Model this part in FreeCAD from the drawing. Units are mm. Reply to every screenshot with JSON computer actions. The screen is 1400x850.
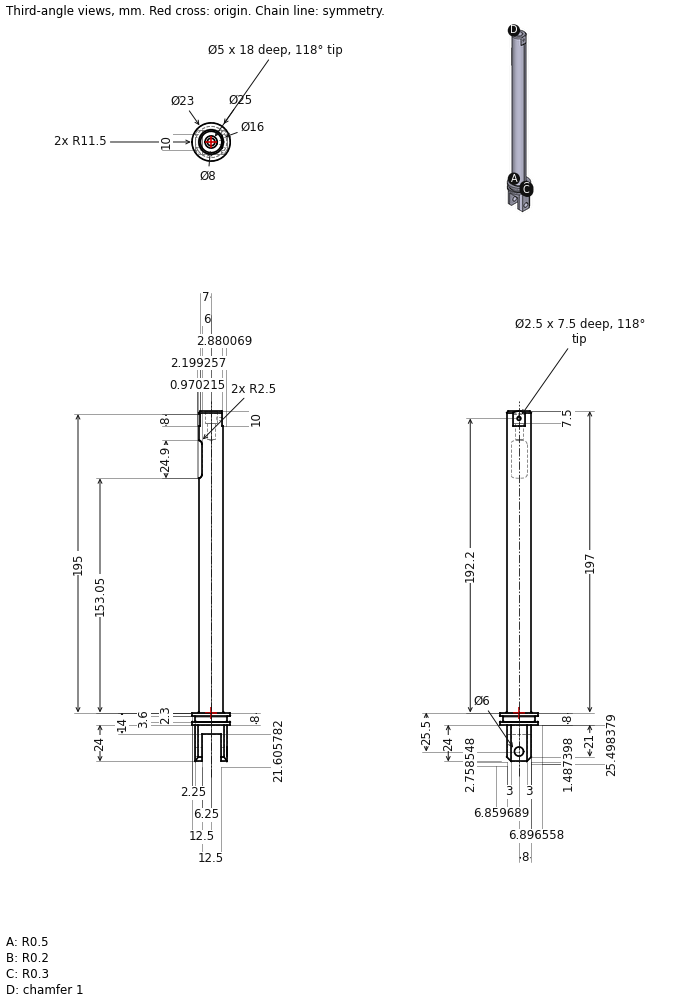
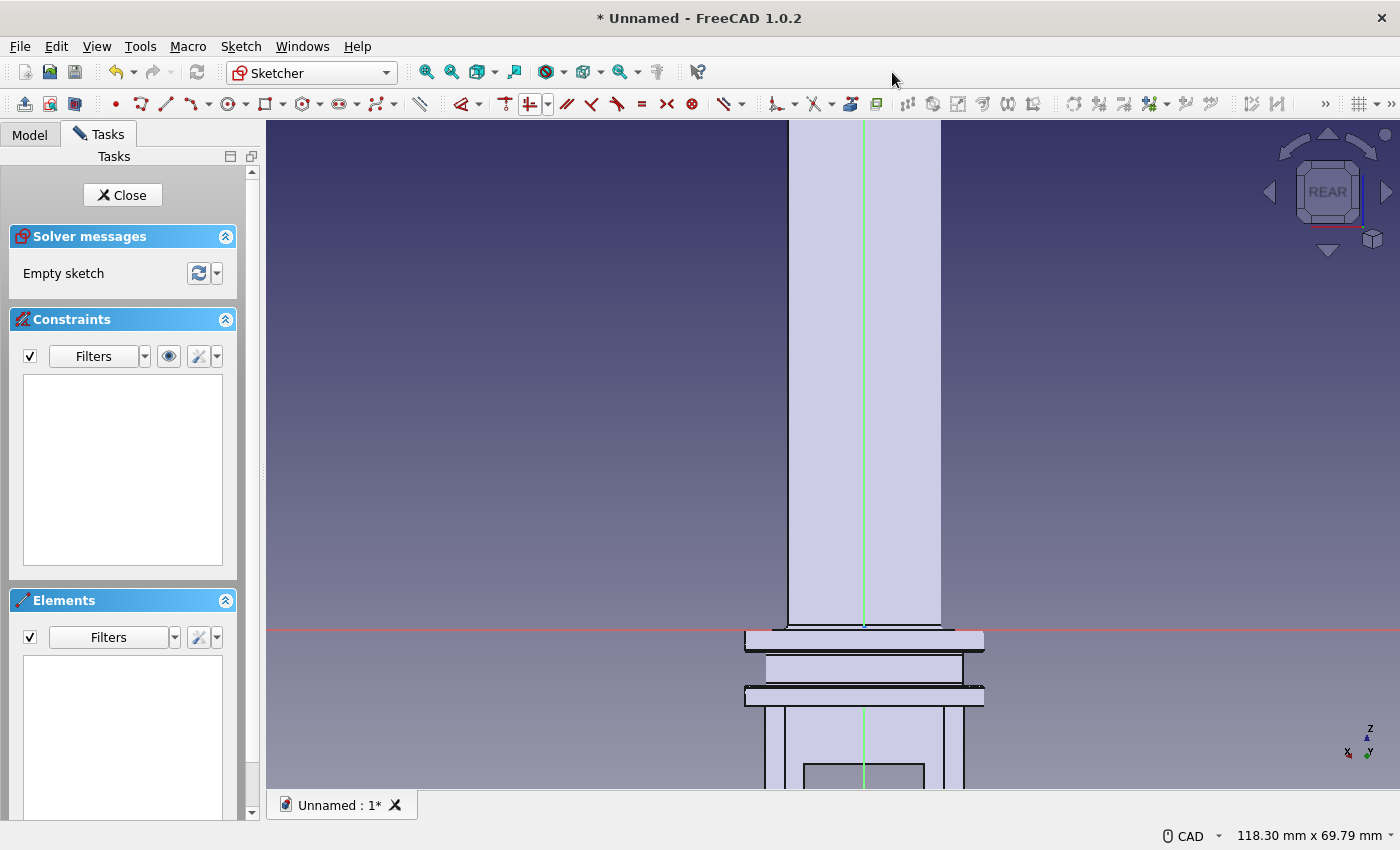
{"action": "scroll", "coordinate": [764, 454], "scroll_direction": "down", "scroll_amount": 5}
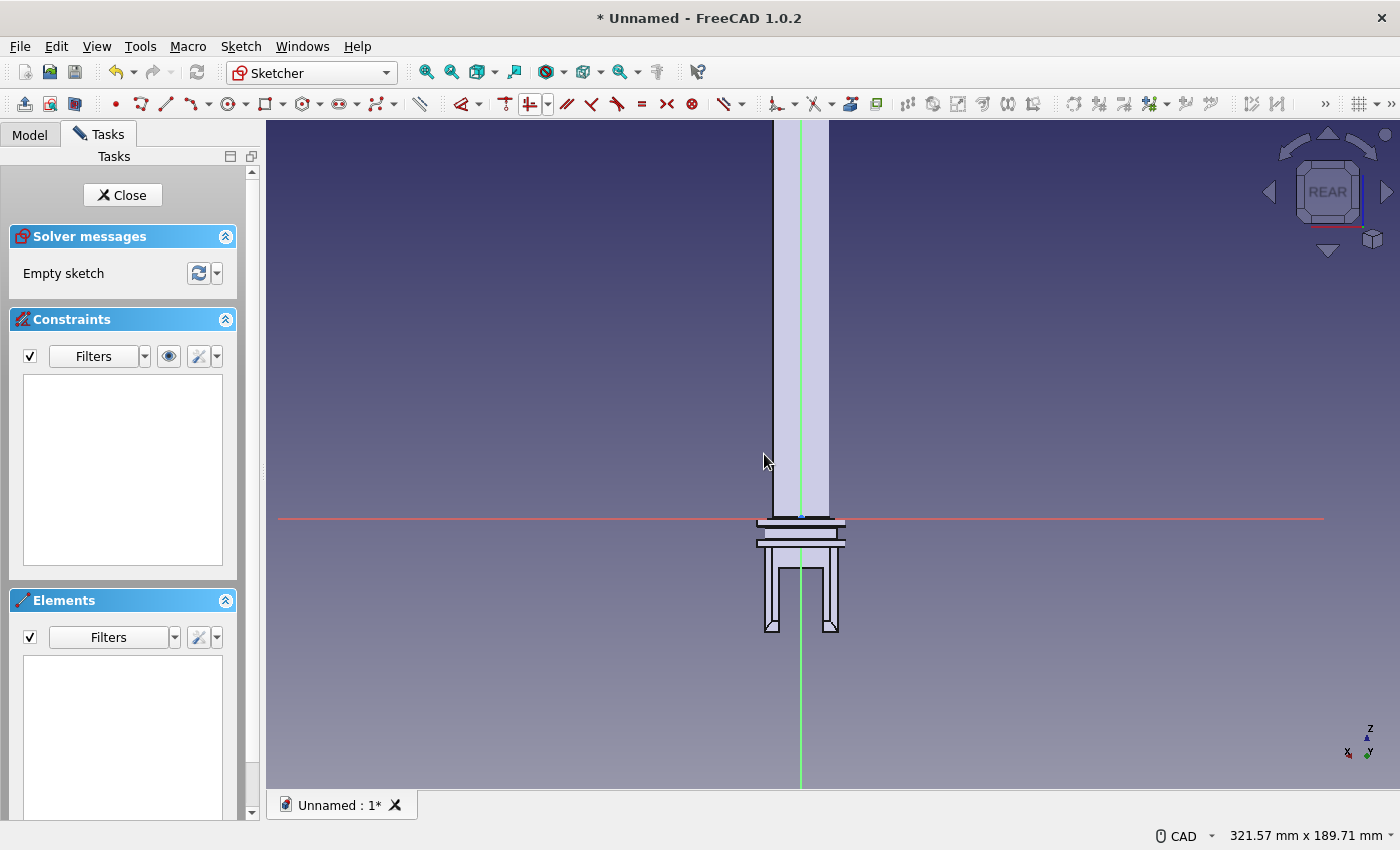
{"action": "scroll", "coordinate": [764, 454], "scroll_direction": "down", "scroll_amount": 5}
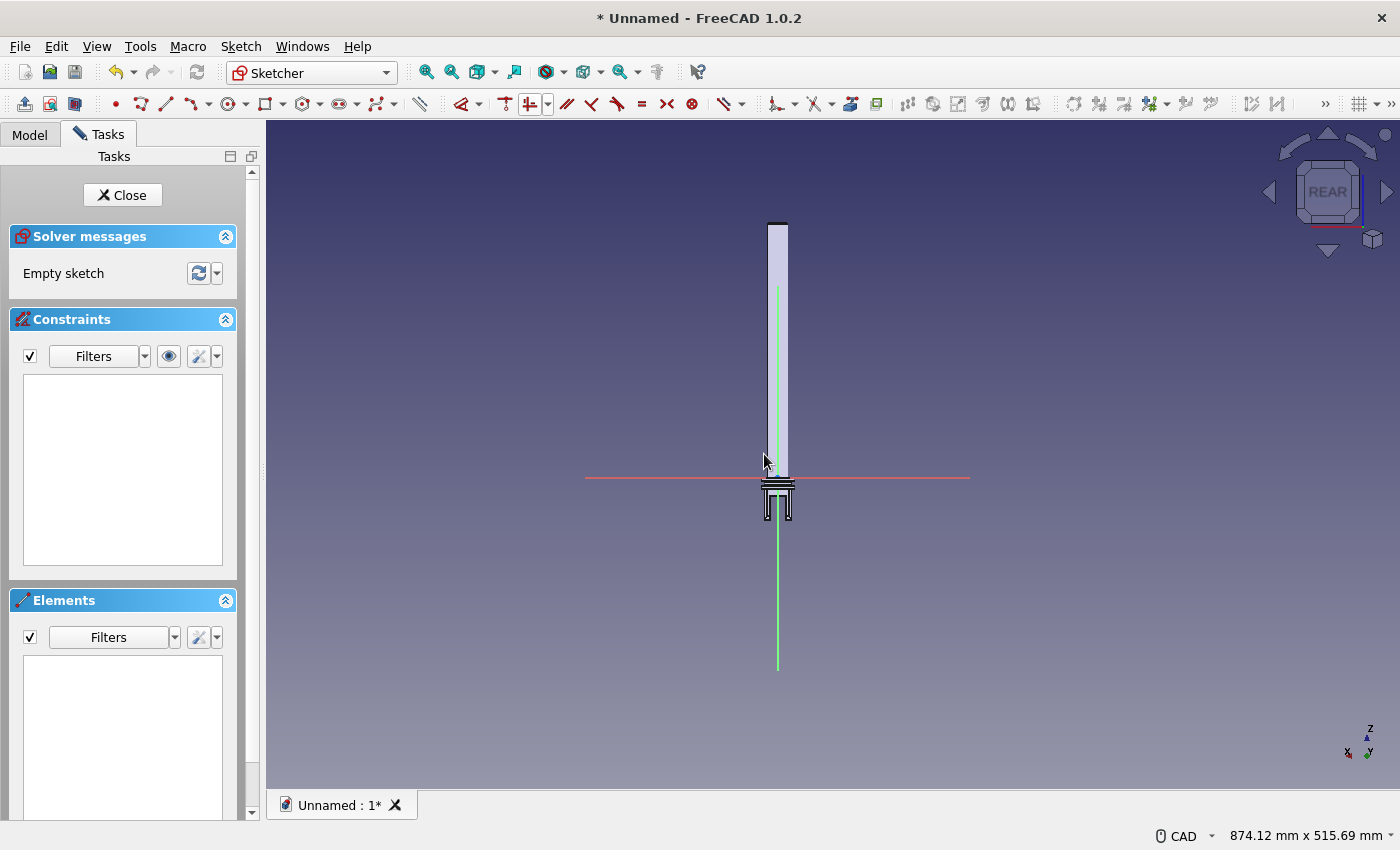
{"action": "scroll", "coordinate": [780, 219], "scroll_direction": "up", "scroll_amount": 10}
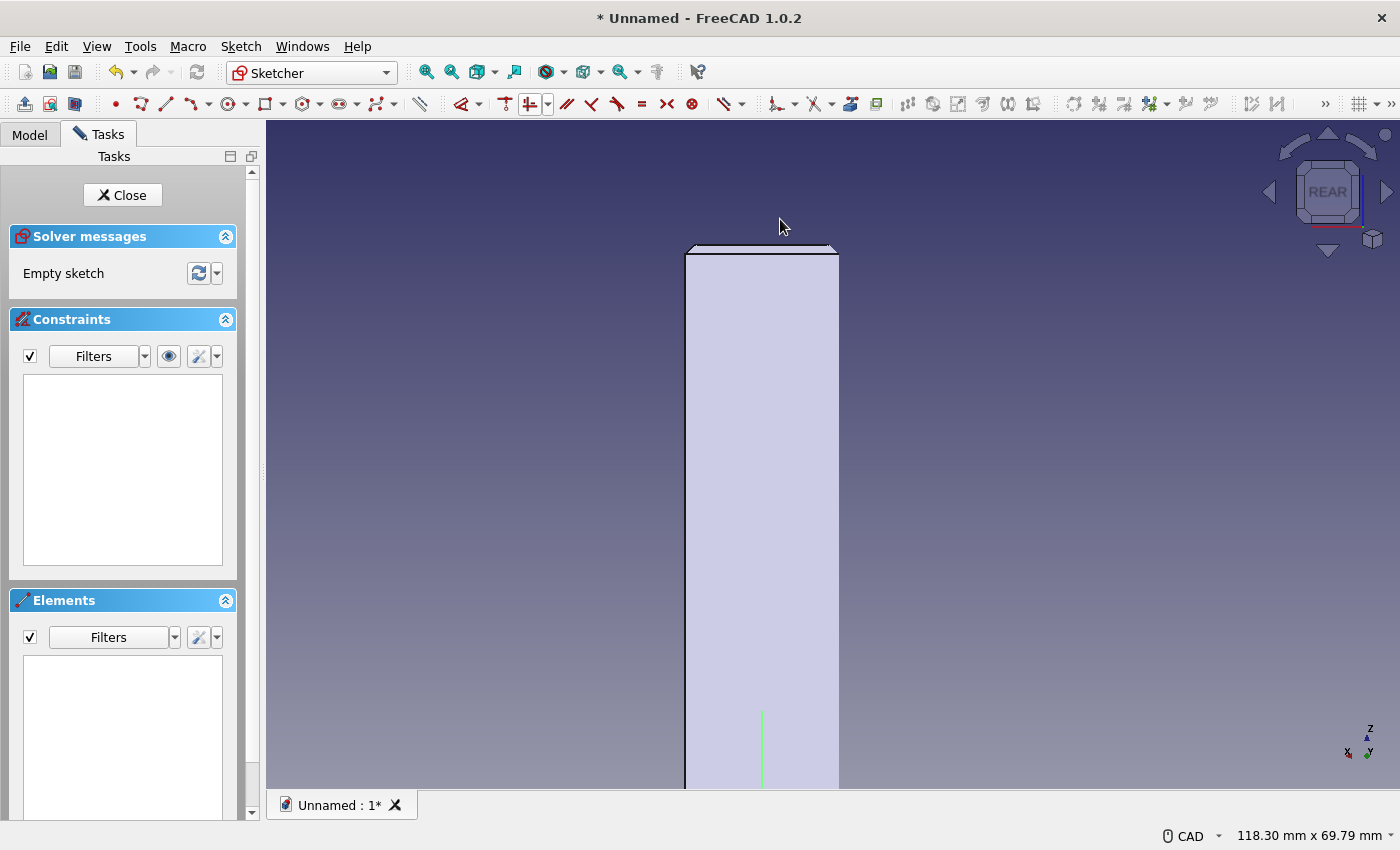
{"action": "left_click", "coordinate": [264, 104]}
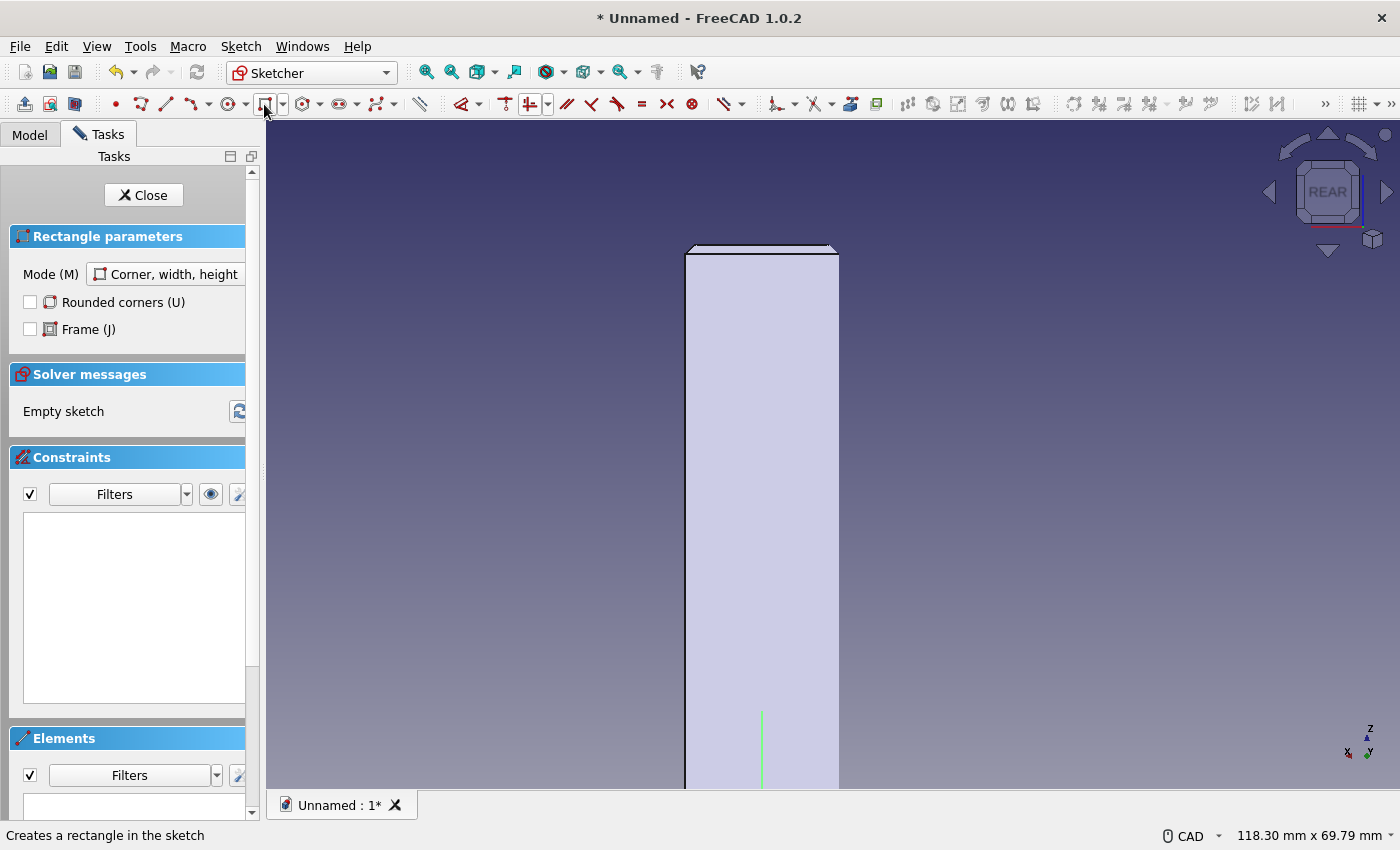
{"action": "left_click", "coordinate": [829, 264]}
{"action": "mouse_move", "coordinate": [850, 341]}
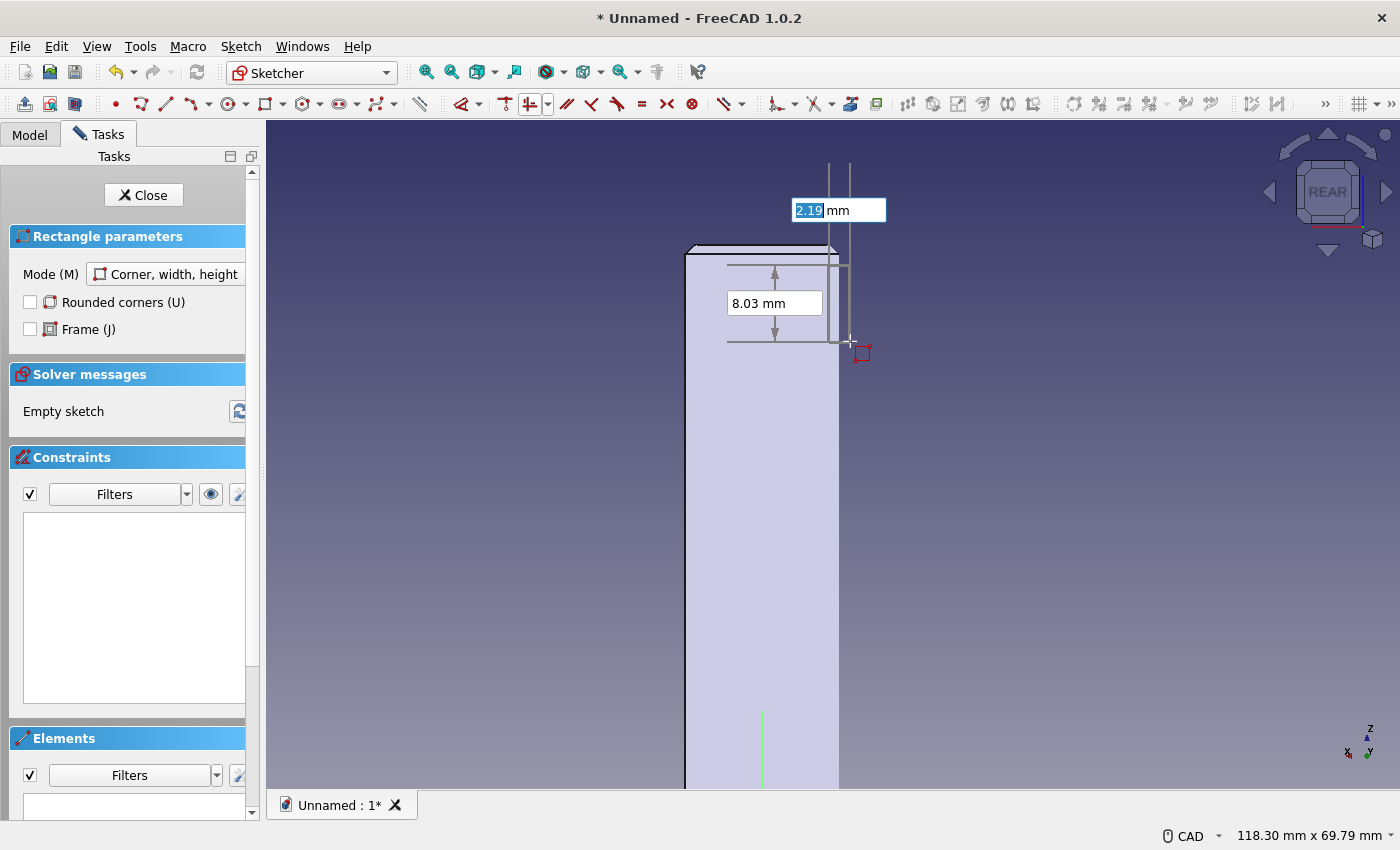
{"action": "type", "text": "2.199257"}
{"action": "key", "text": "Tab"}
{"action": "type", "text": "8"}
{"action": "key", "text": "Return"}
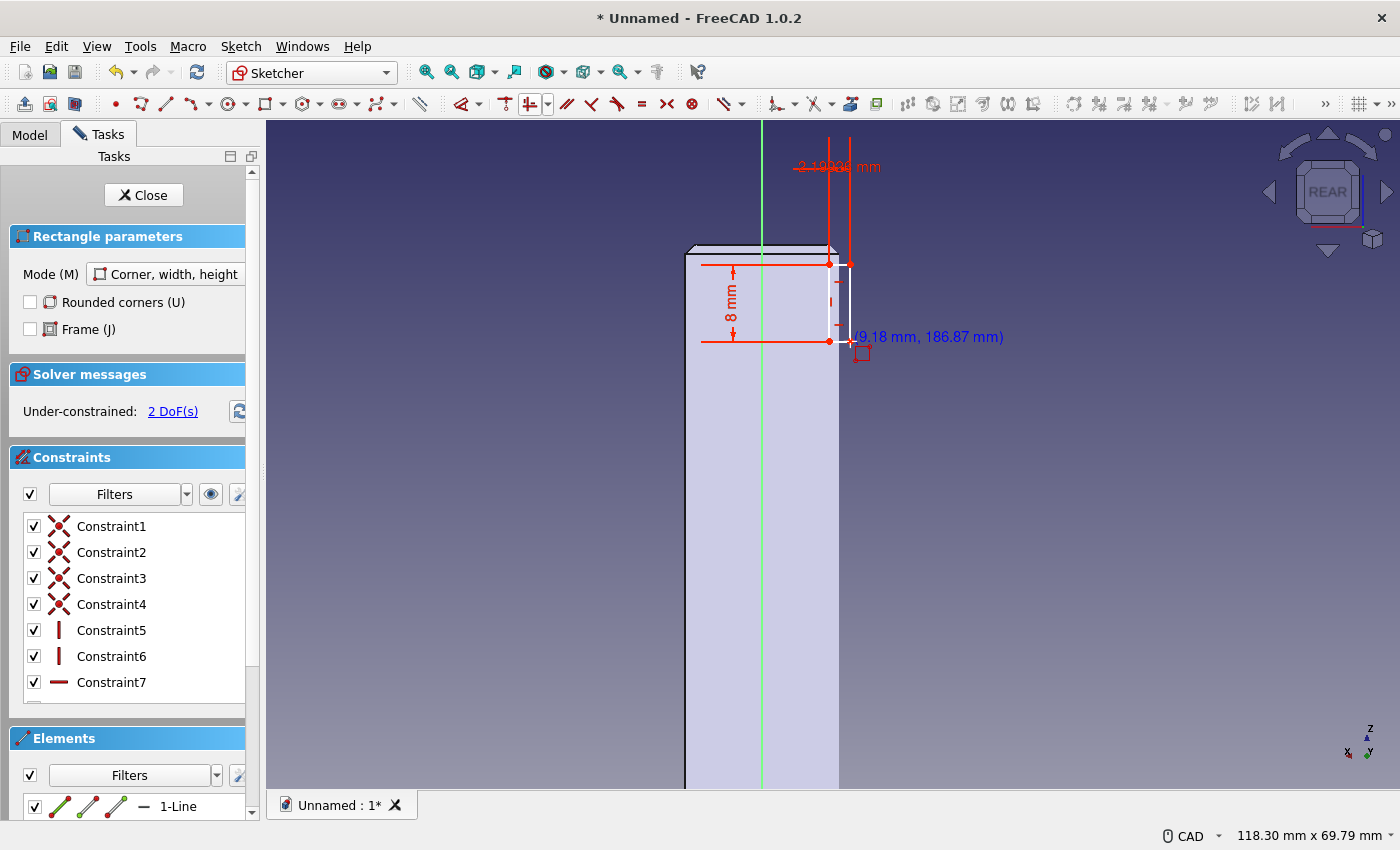
{"action": "left_click", "coordinate": [141, 104]}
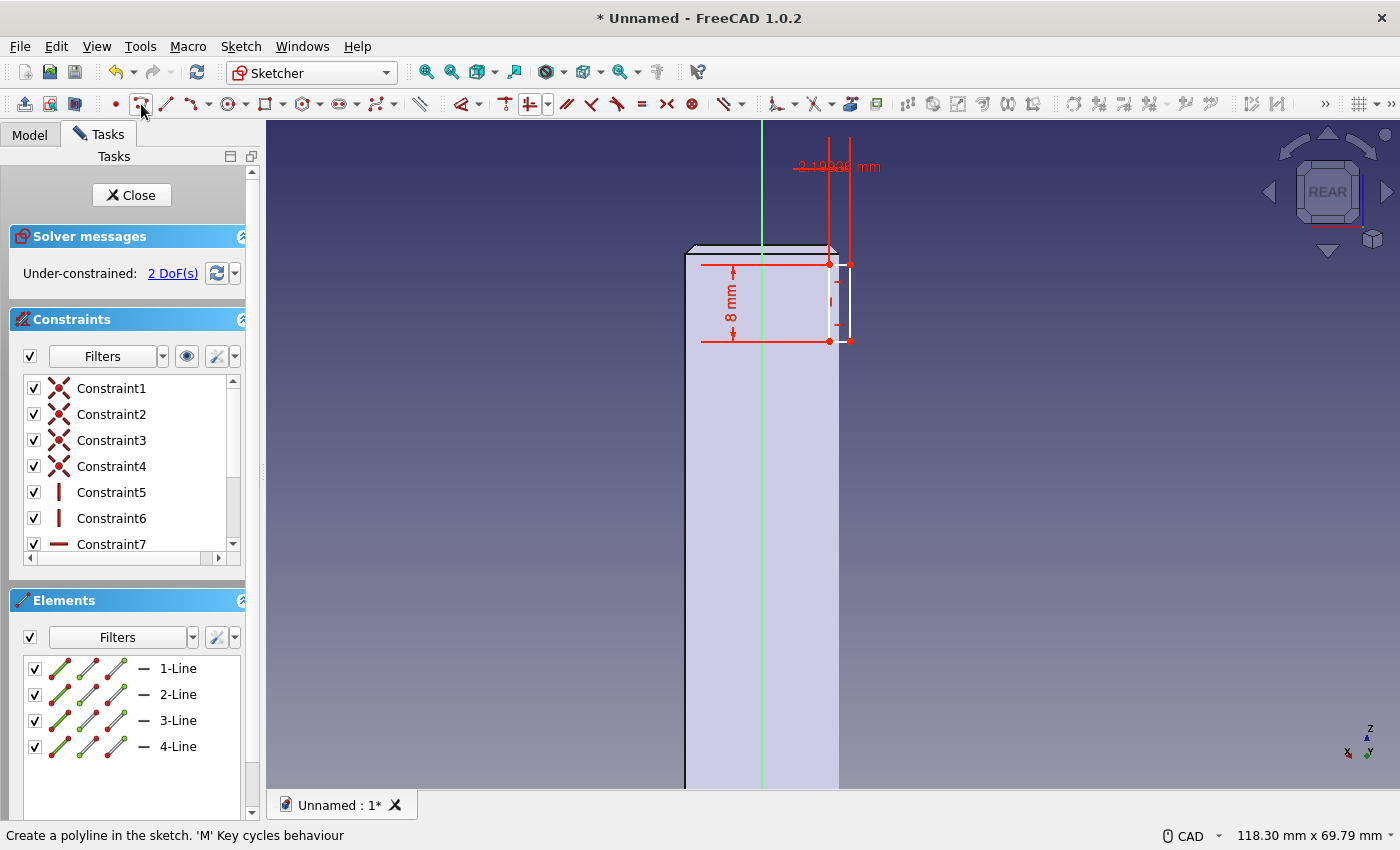
{"action": "left_click", "coordinate": [844, 666]}